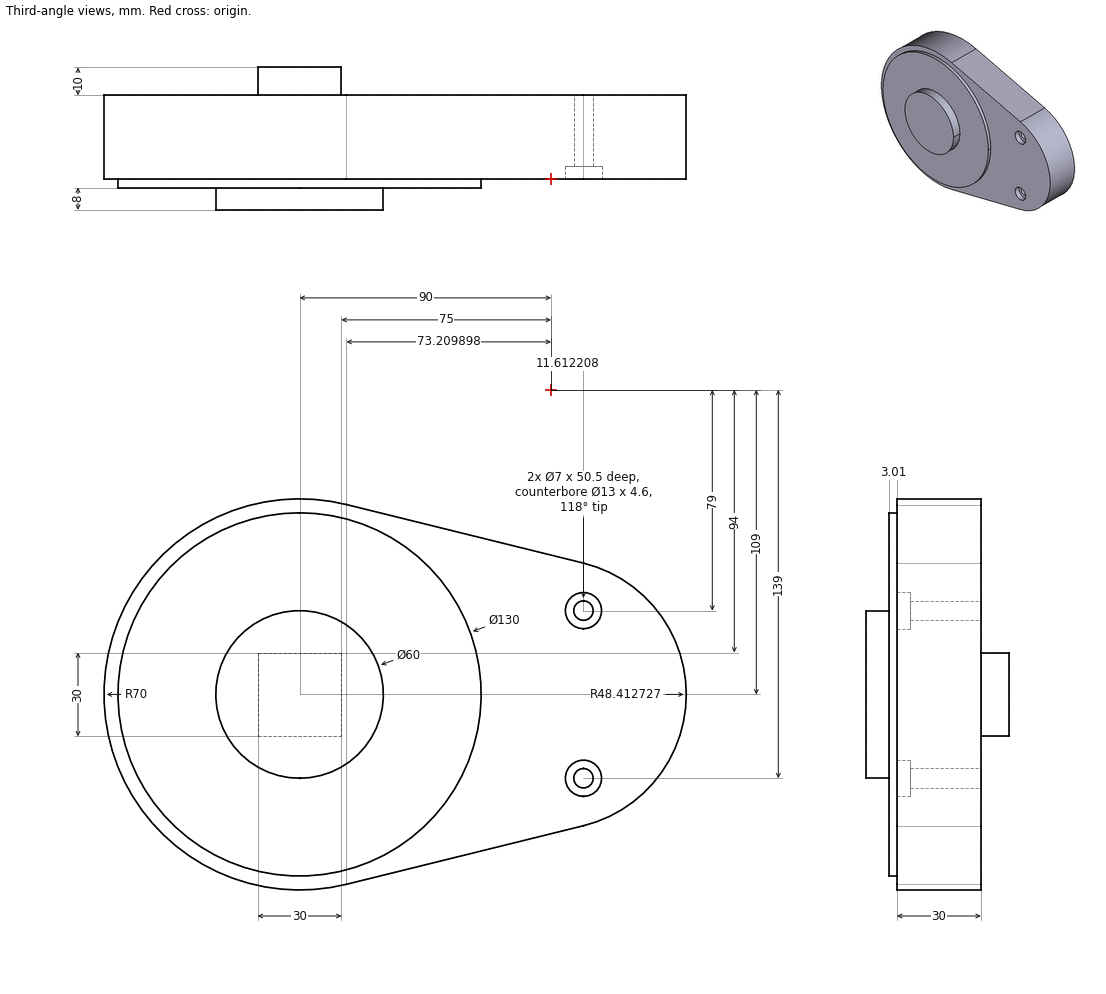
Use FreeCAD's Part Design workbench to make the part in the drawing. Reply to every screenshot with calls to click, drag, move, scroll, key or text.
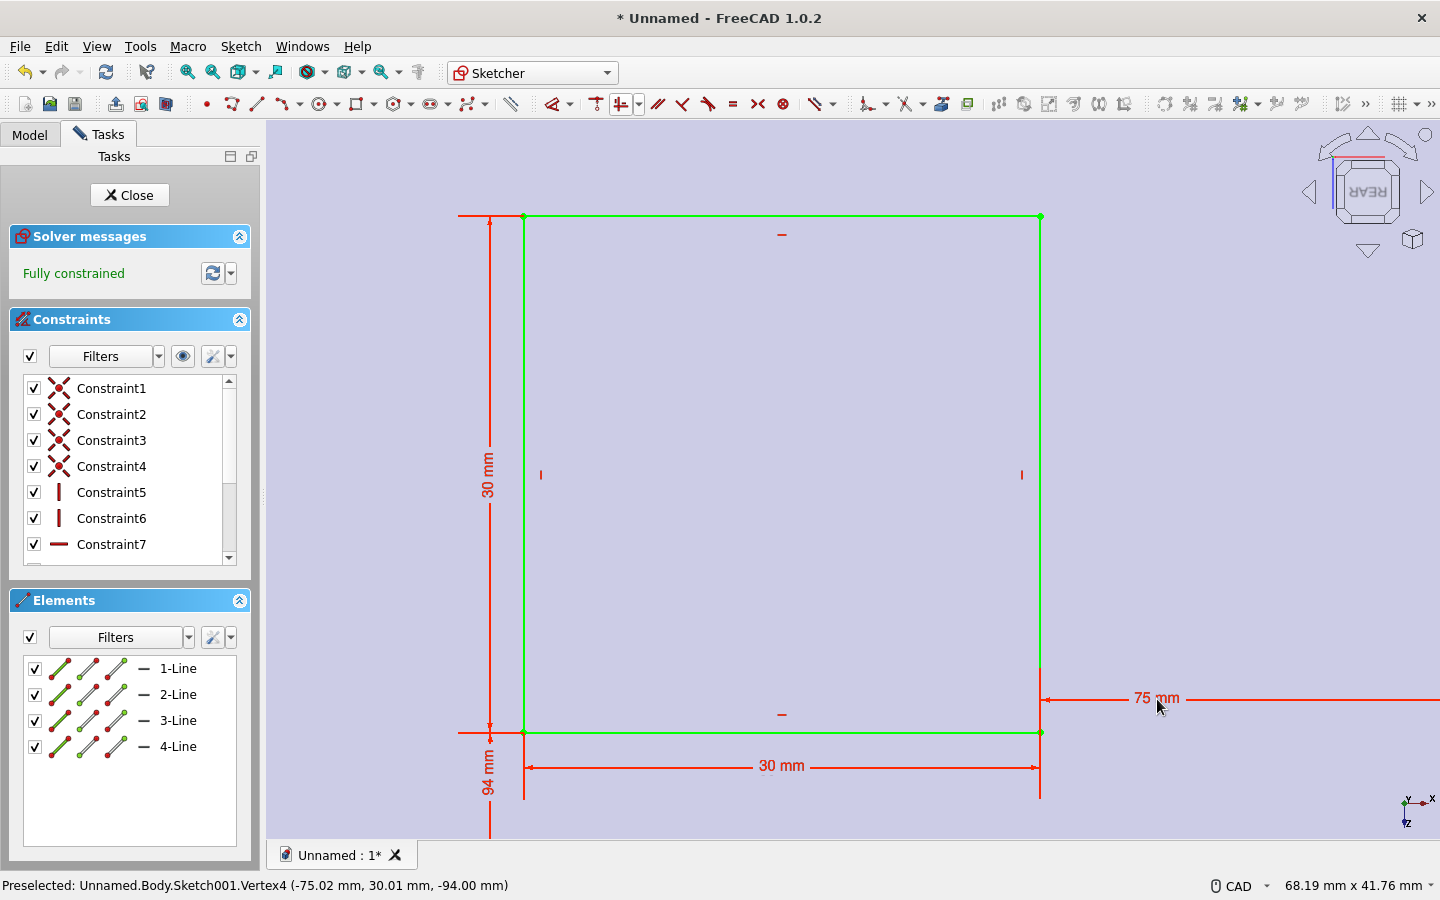
click(130, 195)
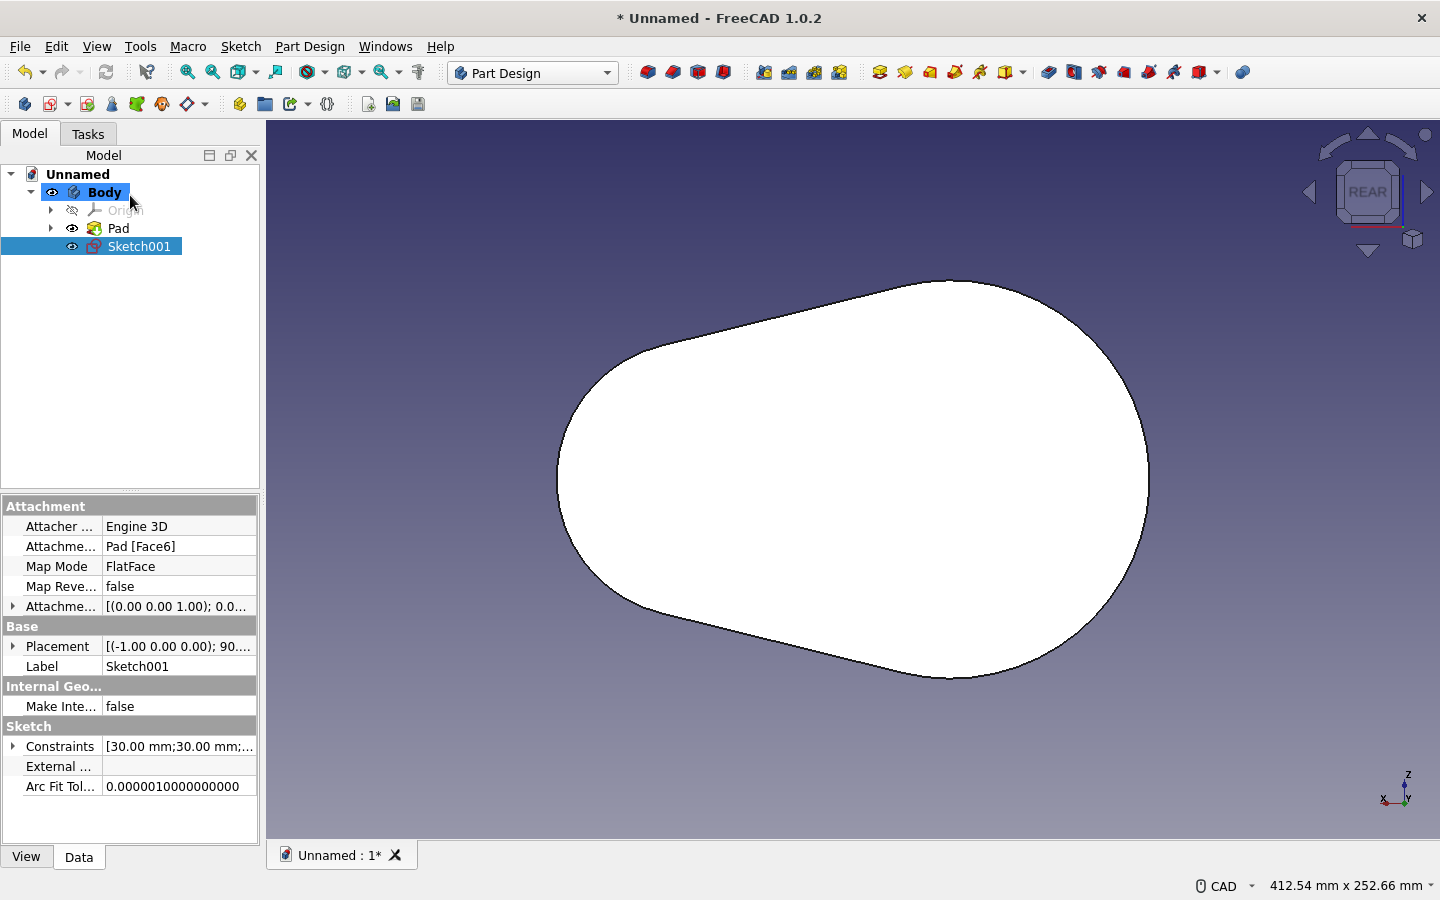
click(880, 72)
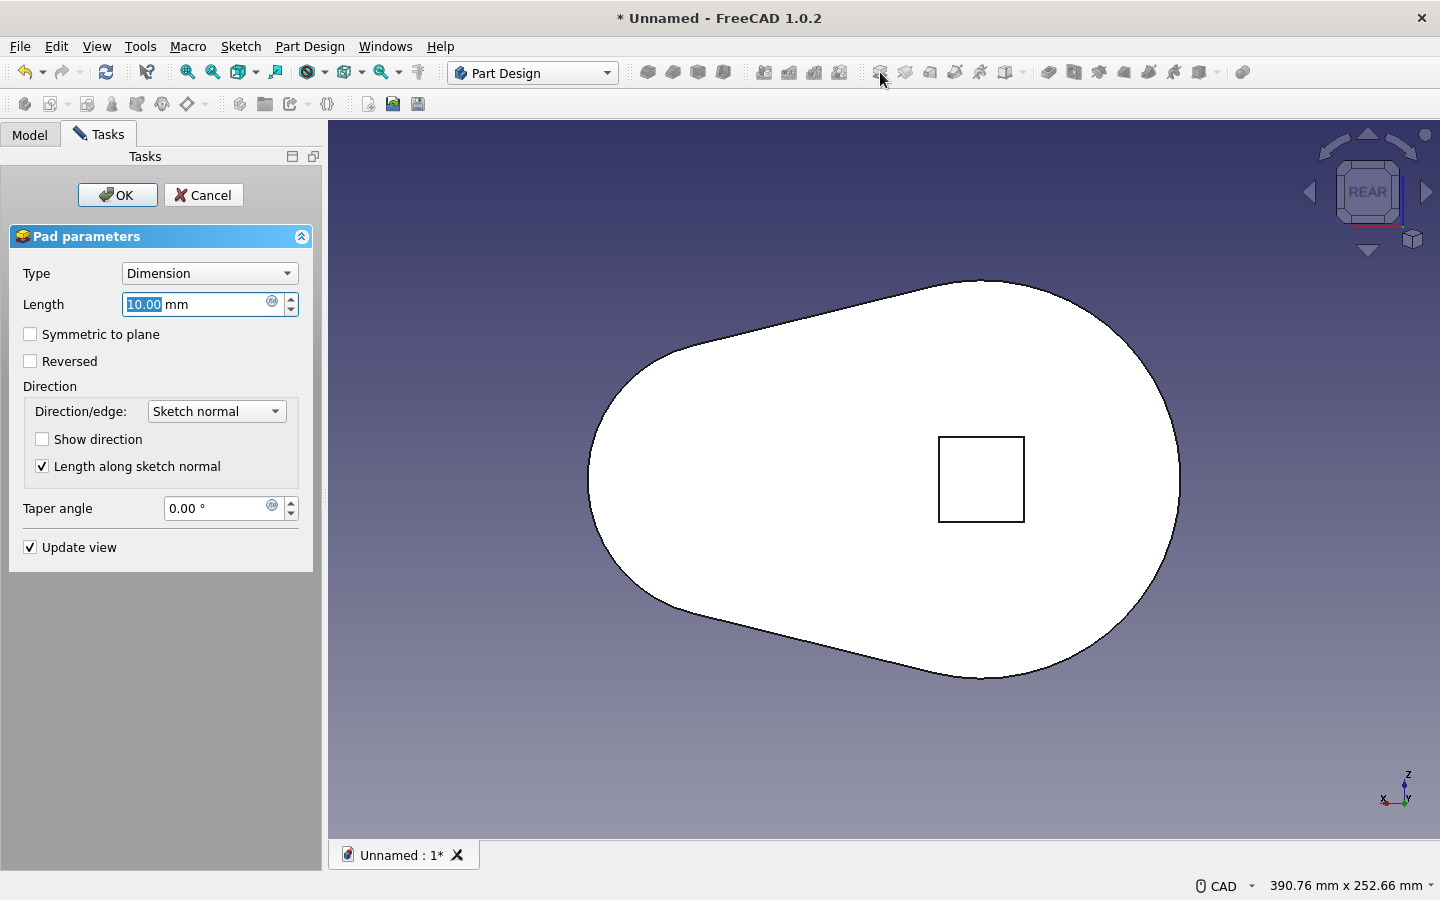
text(10)
key(Tab)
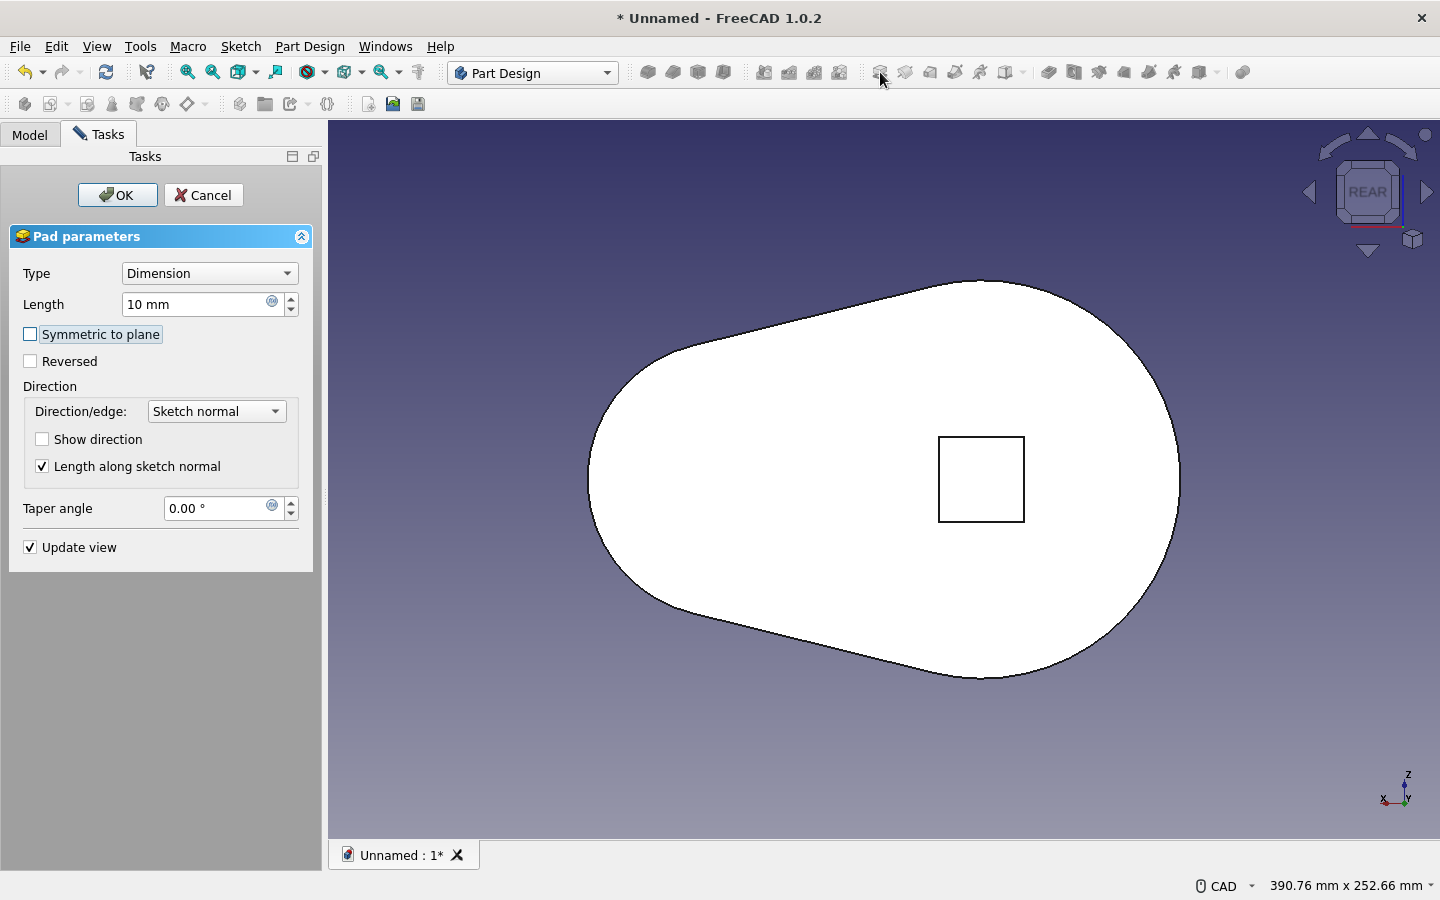
click(118, 195)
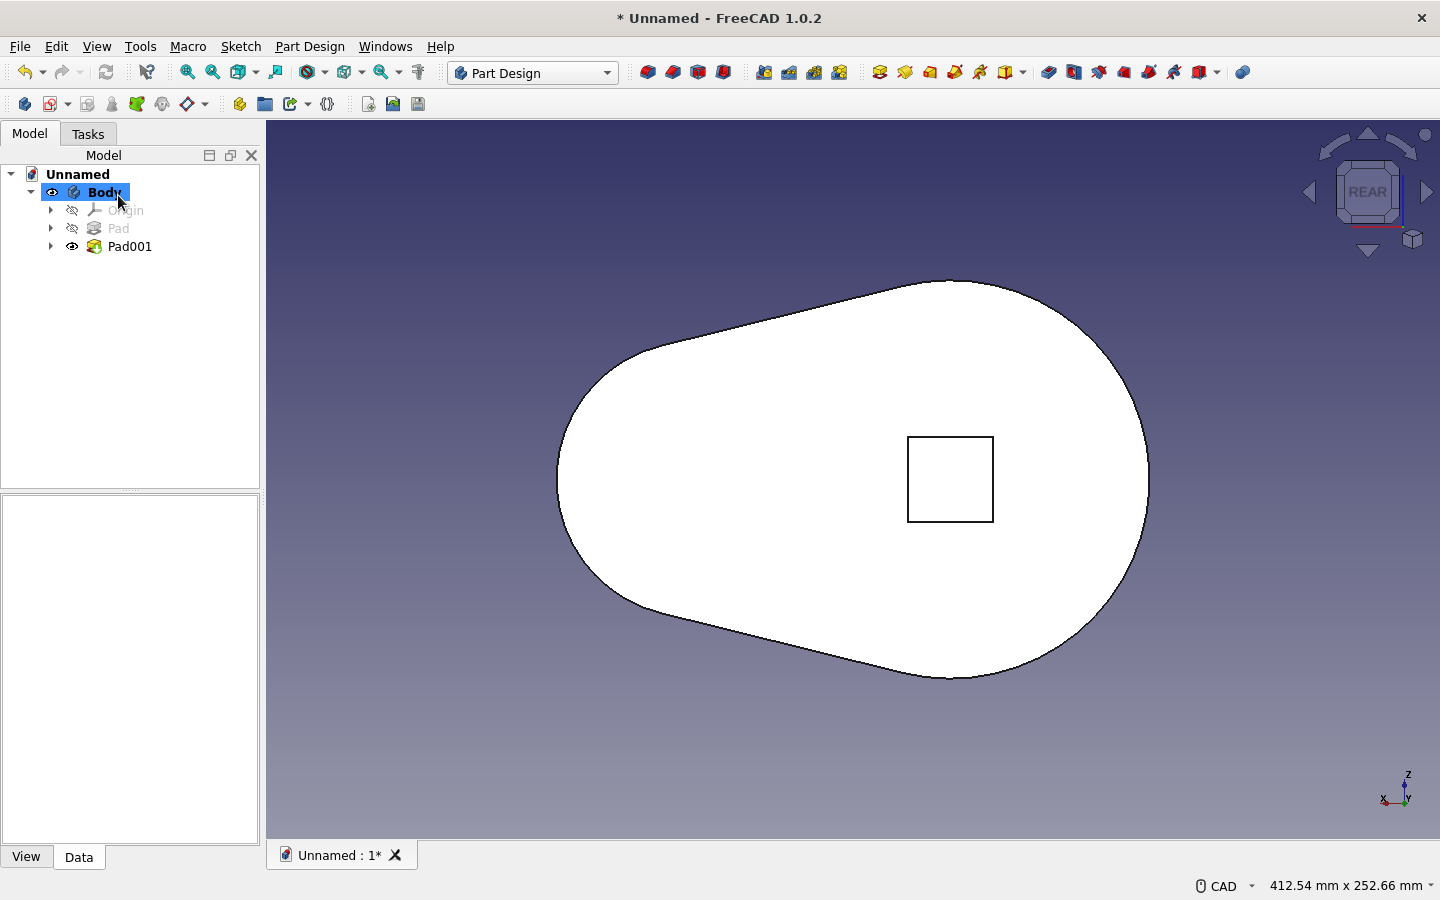
key(0)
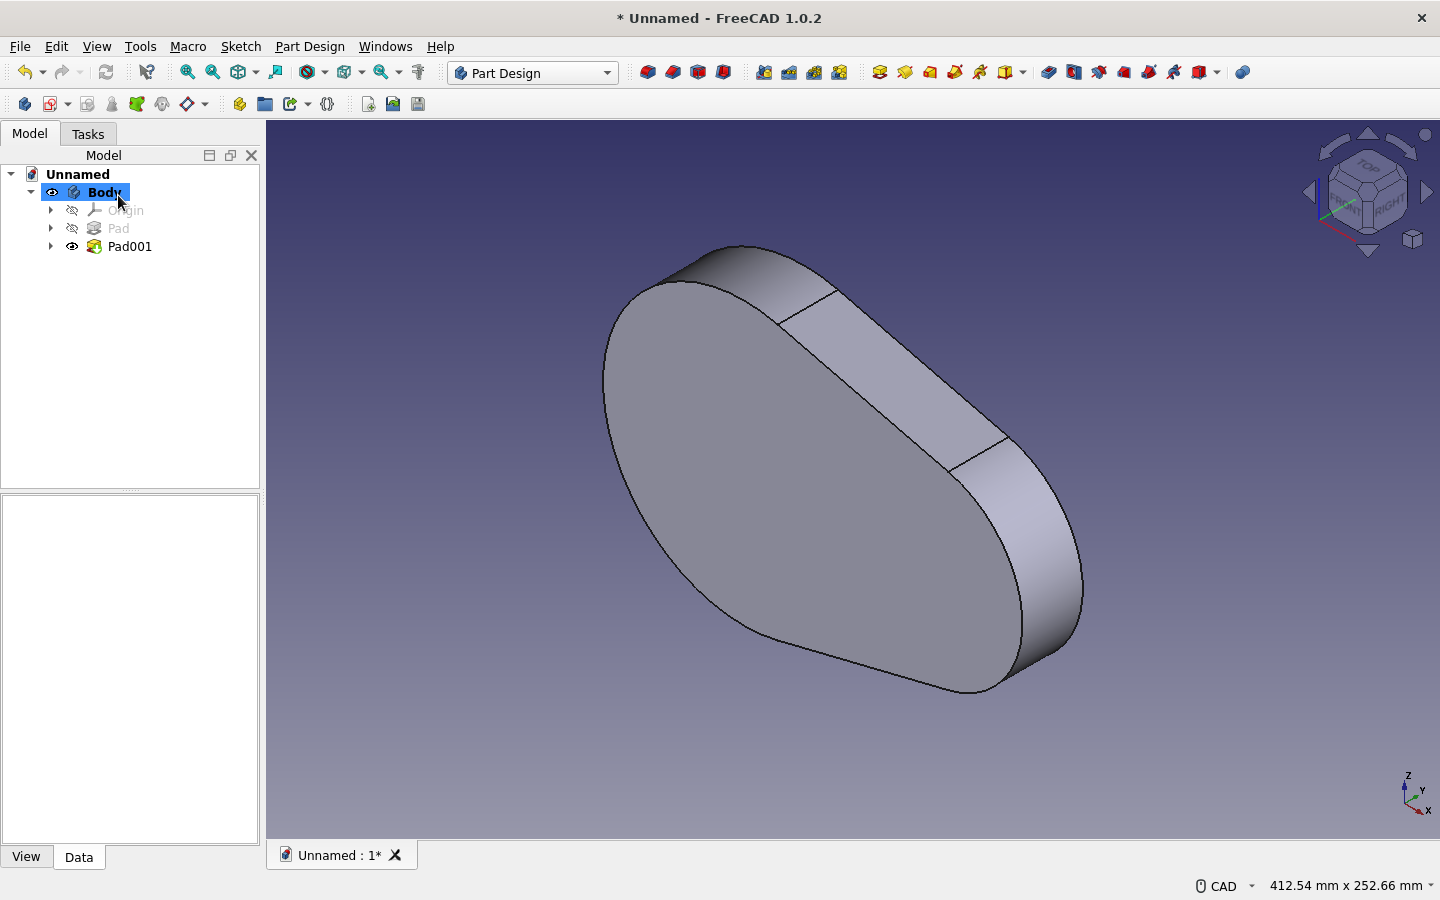
click(753, 467)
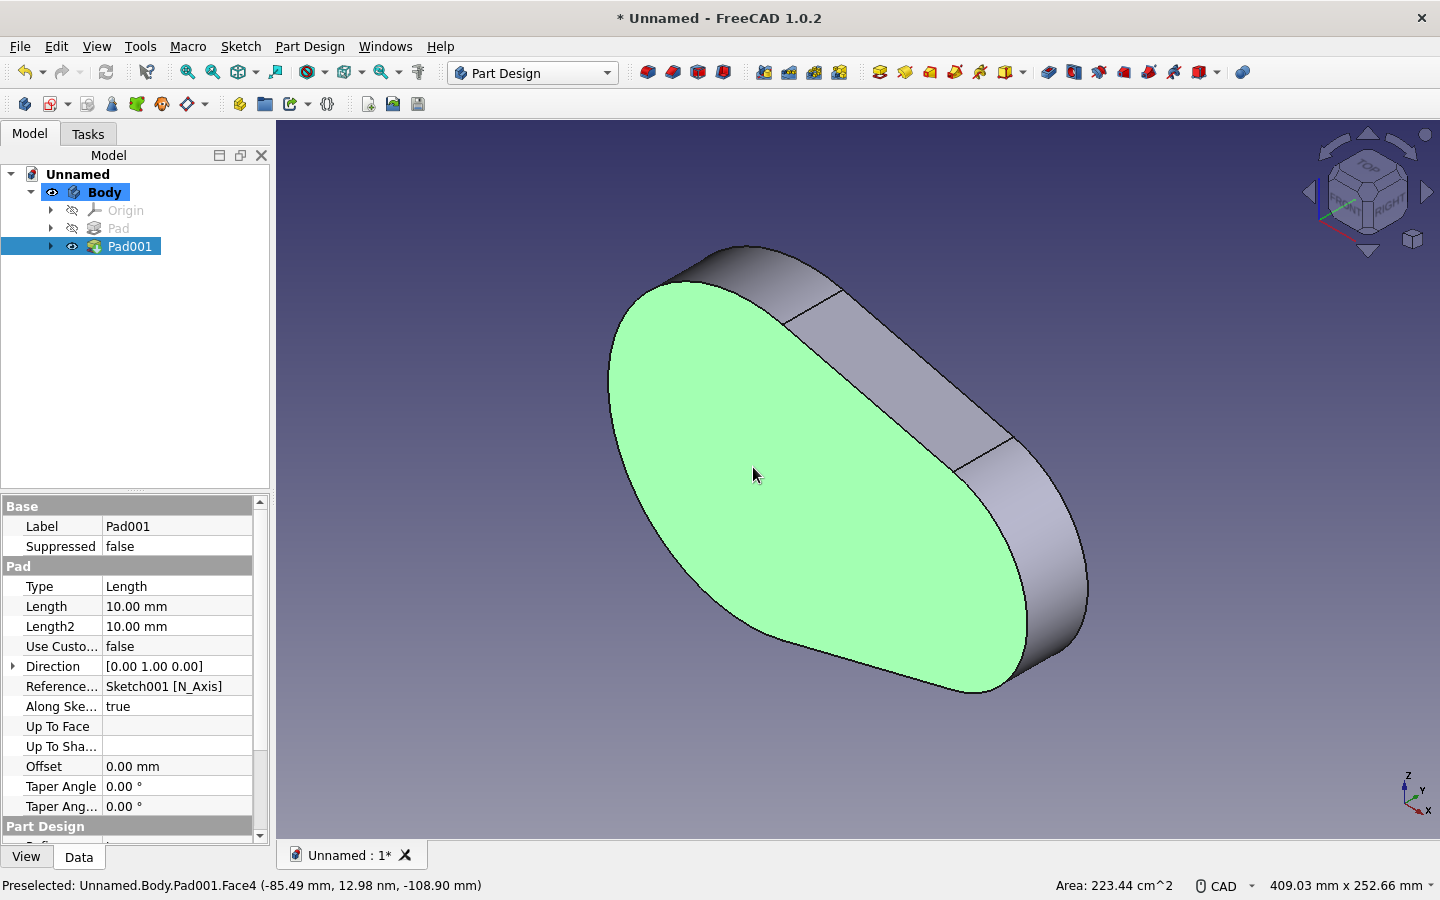
click(50, 104)